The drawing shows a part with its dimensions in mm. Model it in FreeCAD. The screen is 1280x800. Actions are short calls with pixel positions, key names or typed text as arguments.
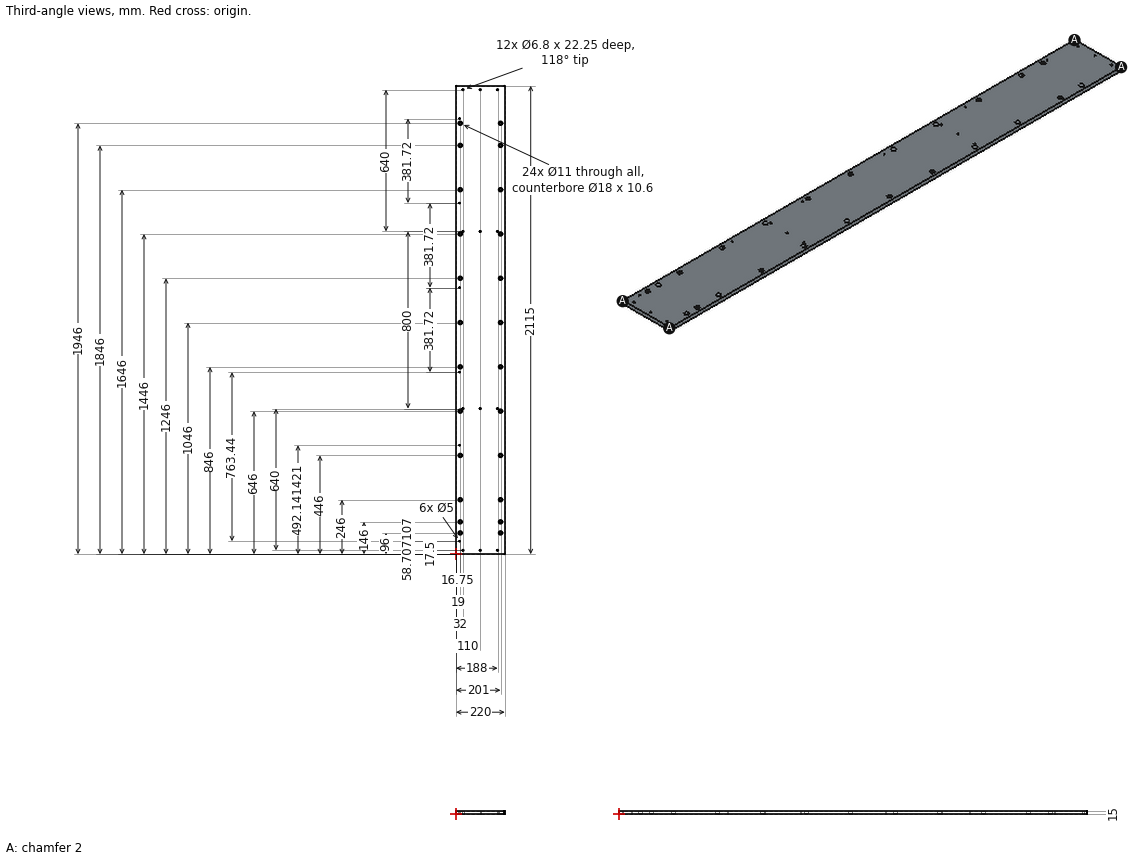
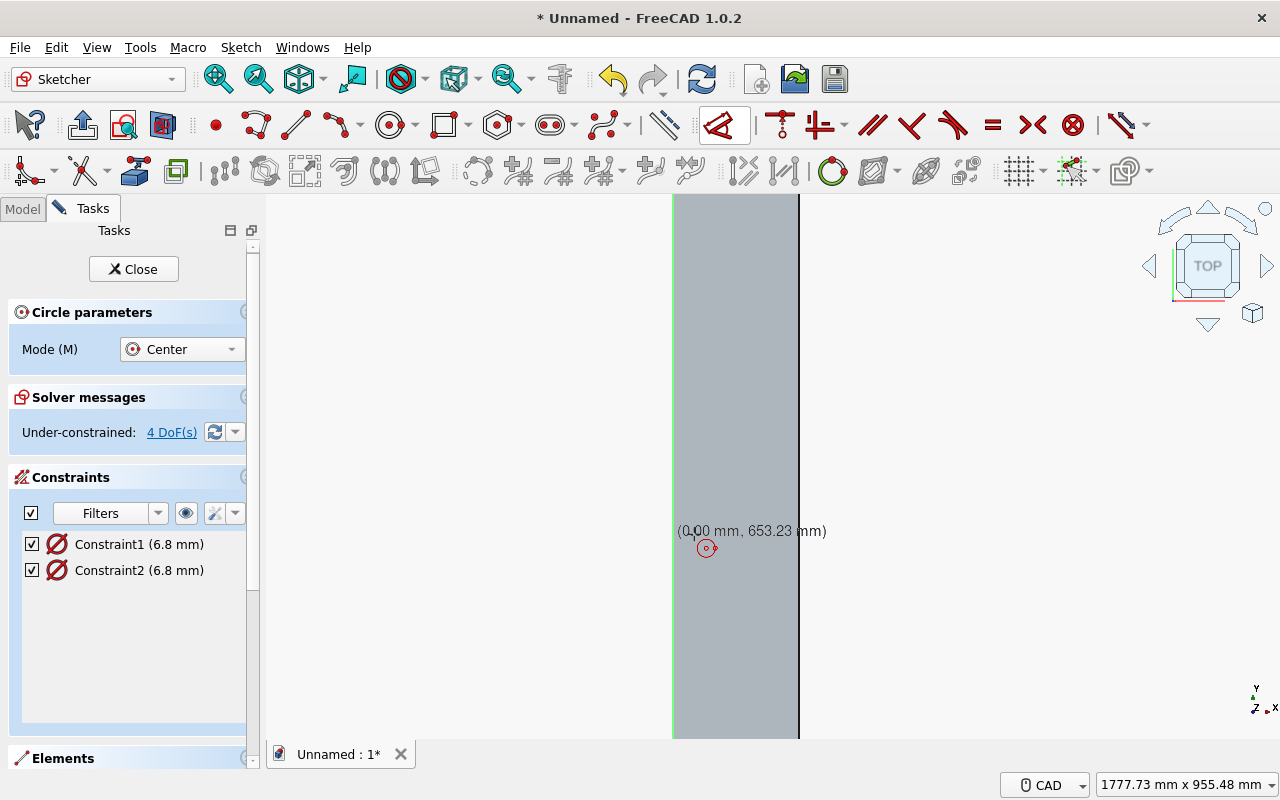
click(692, 533)
move(693, 532)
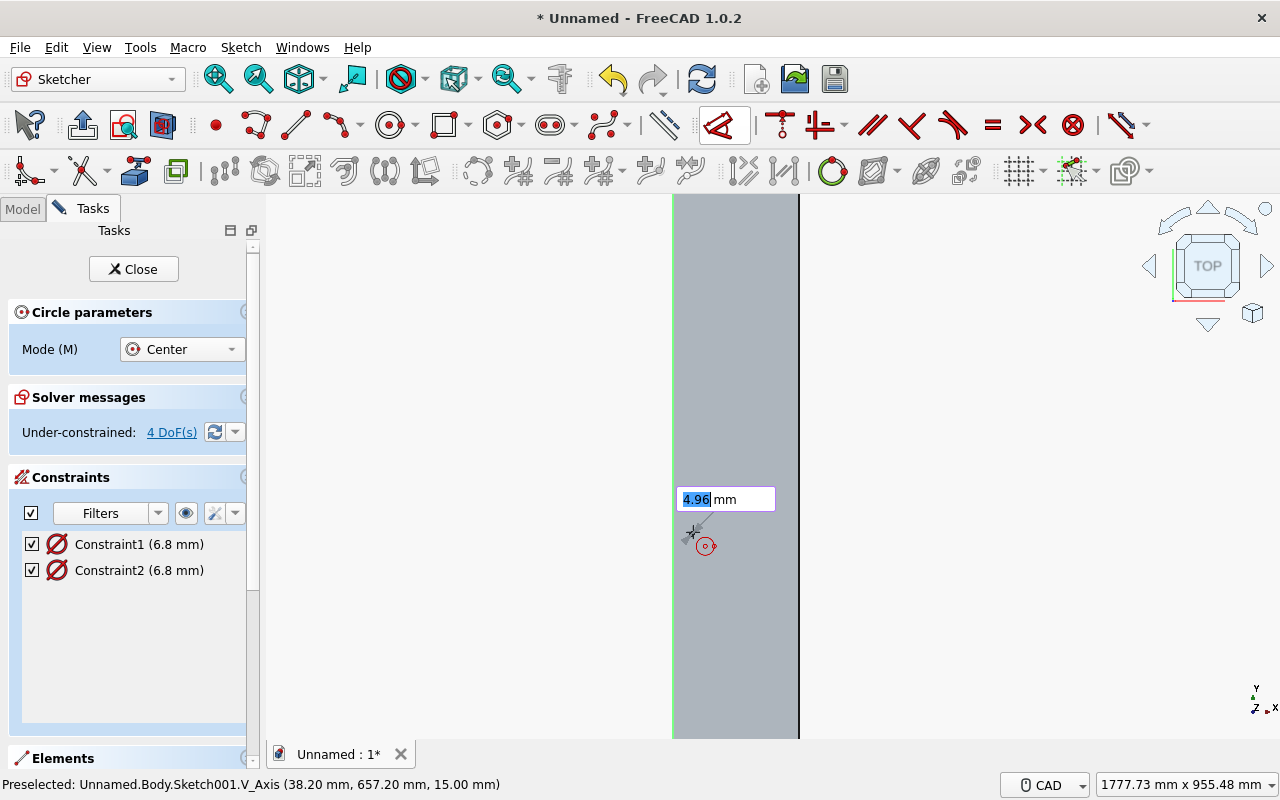
text(6.8)
key(Return)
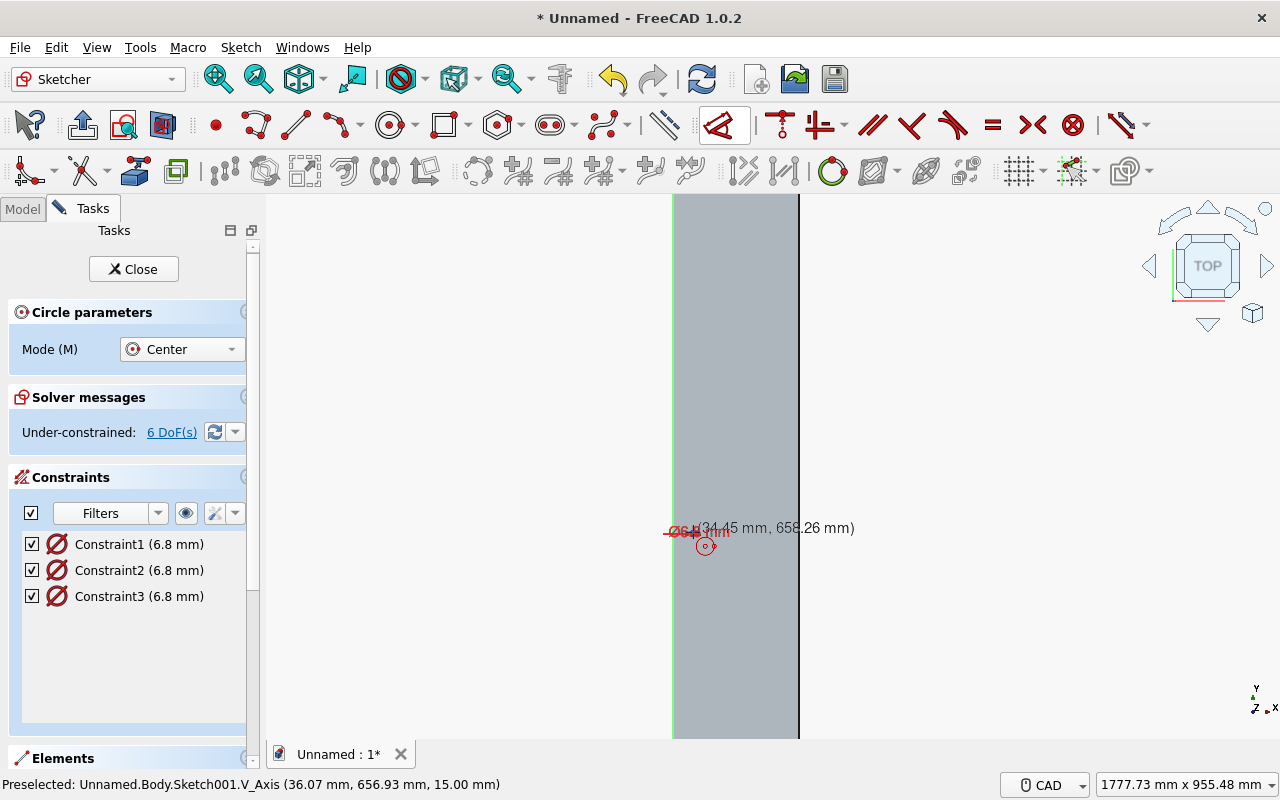
scroll(694, 534, down, 6)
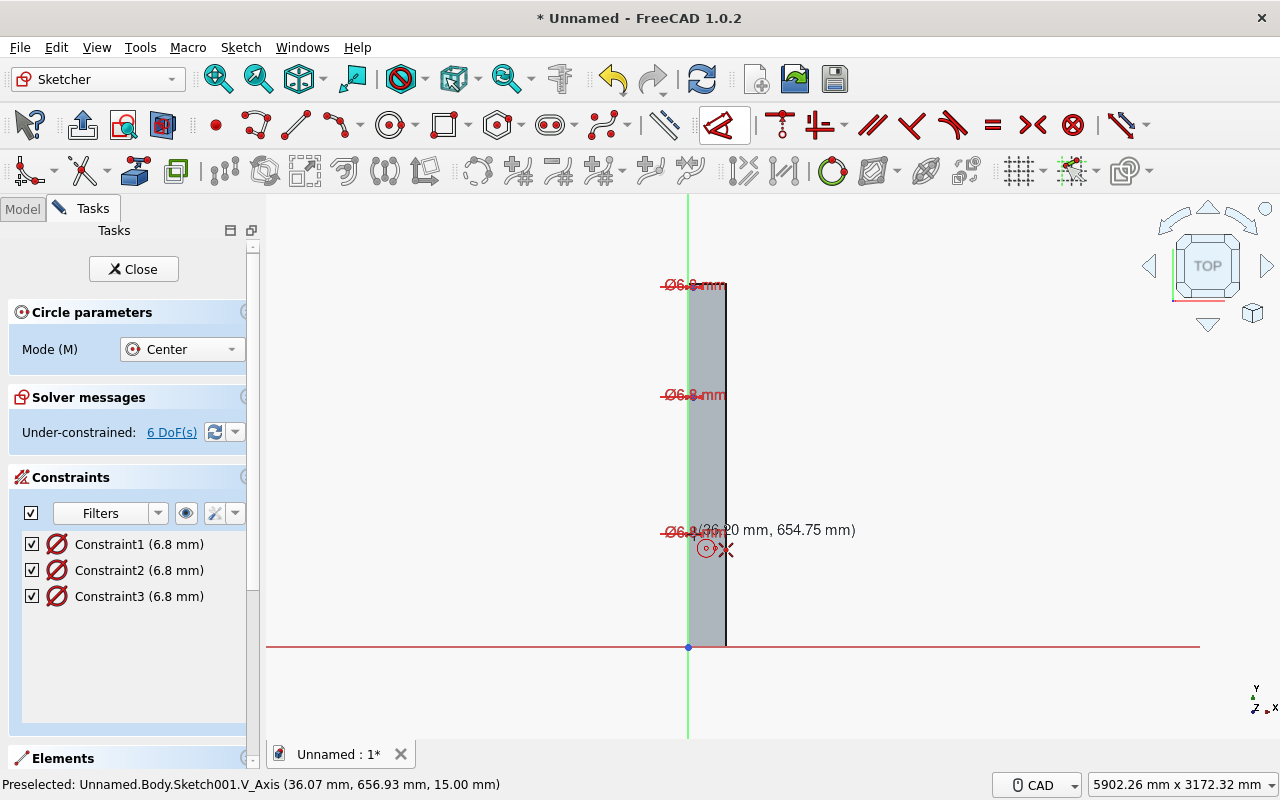
scroll(694, 644, up, 19)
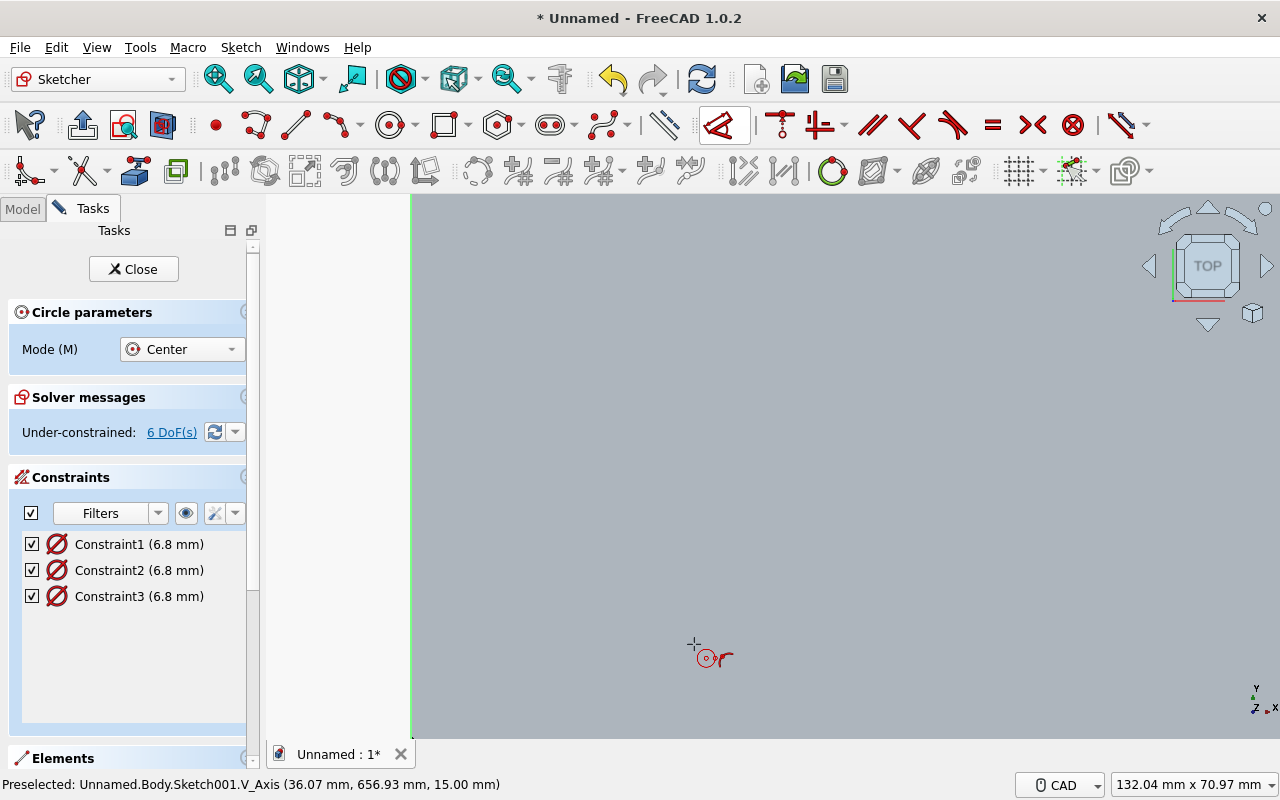
scroll(704, 466, down, 15)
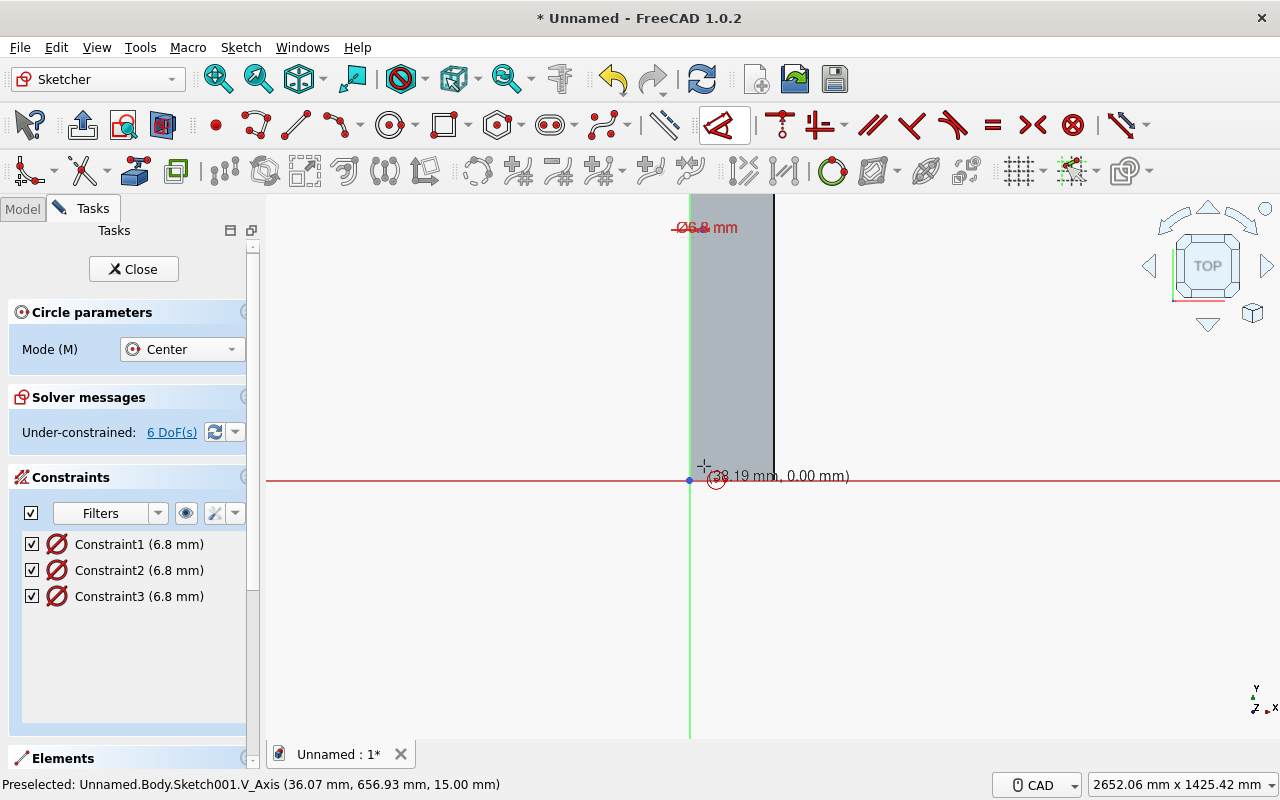
scroll(692, 692, down, 5)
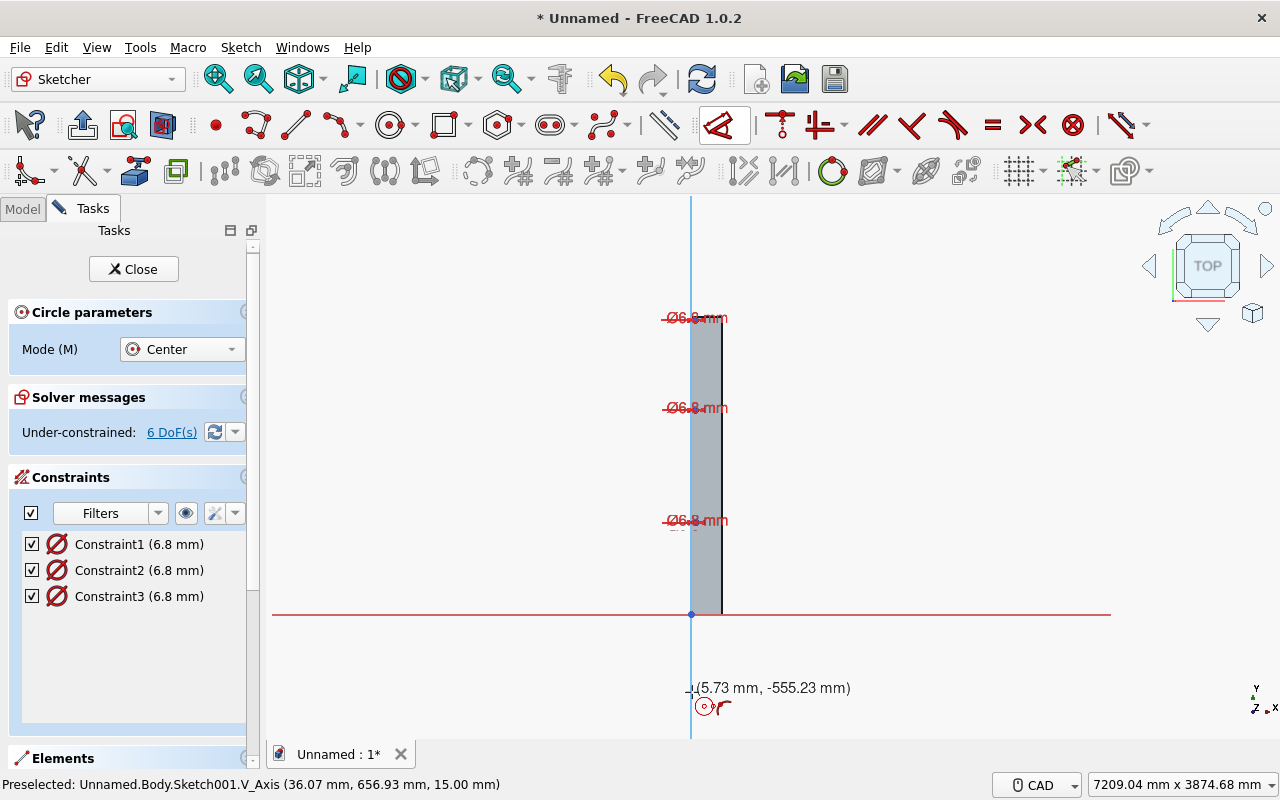
scroll(696, 612, up, 10)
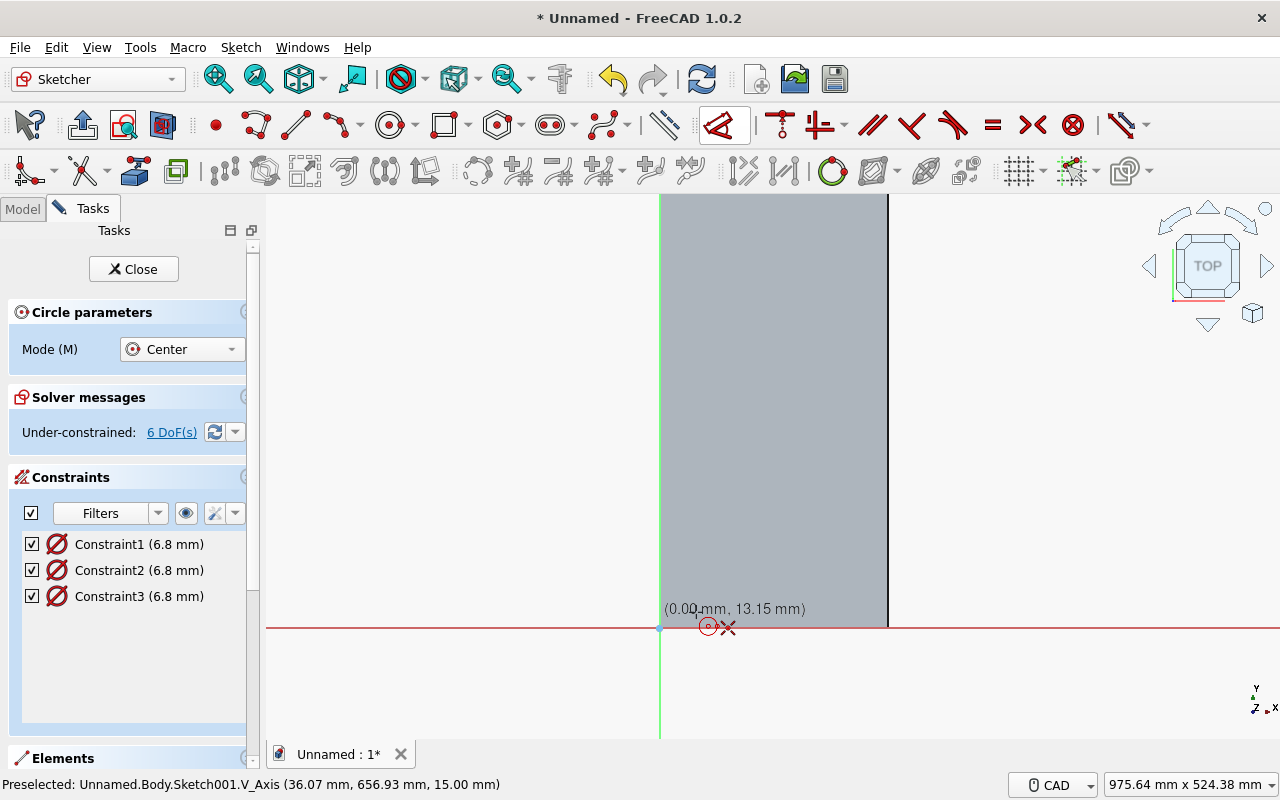
click(693, 610)
move(695, 607)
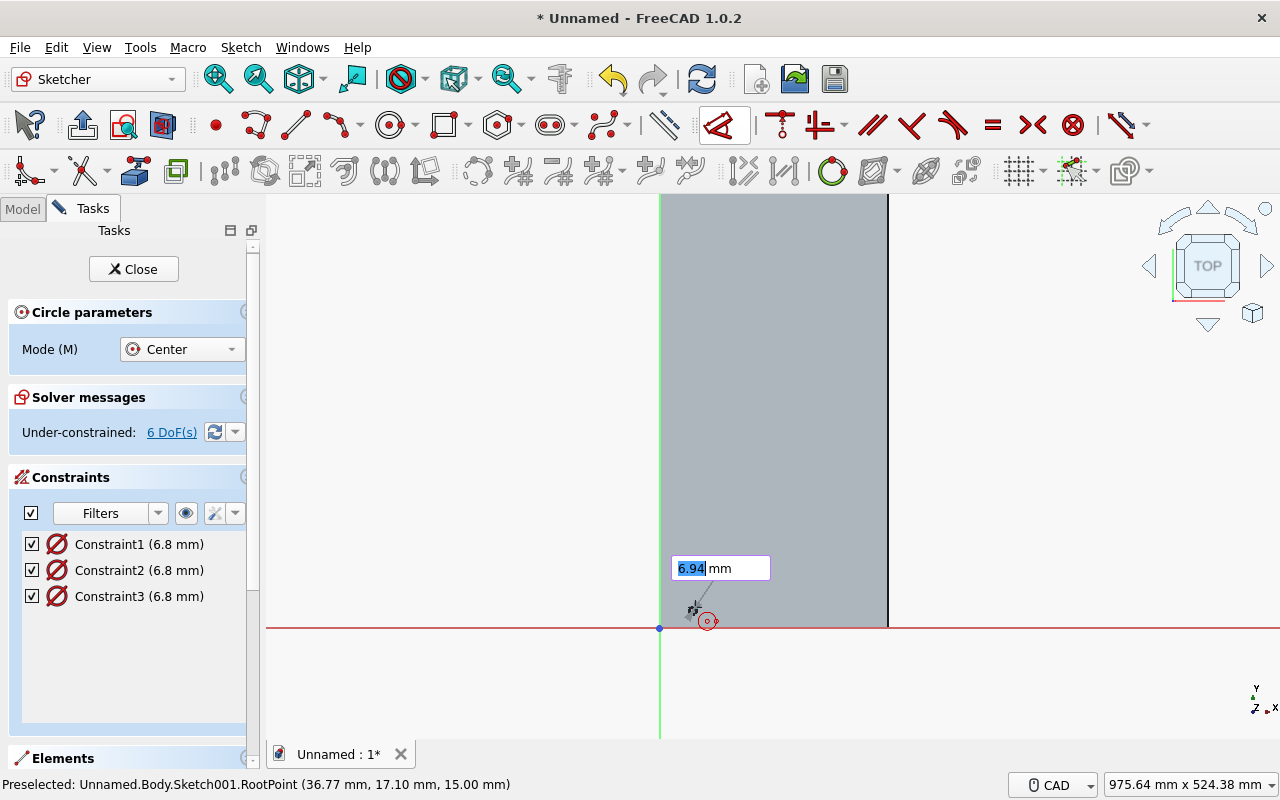
text(6.8)
key(Return)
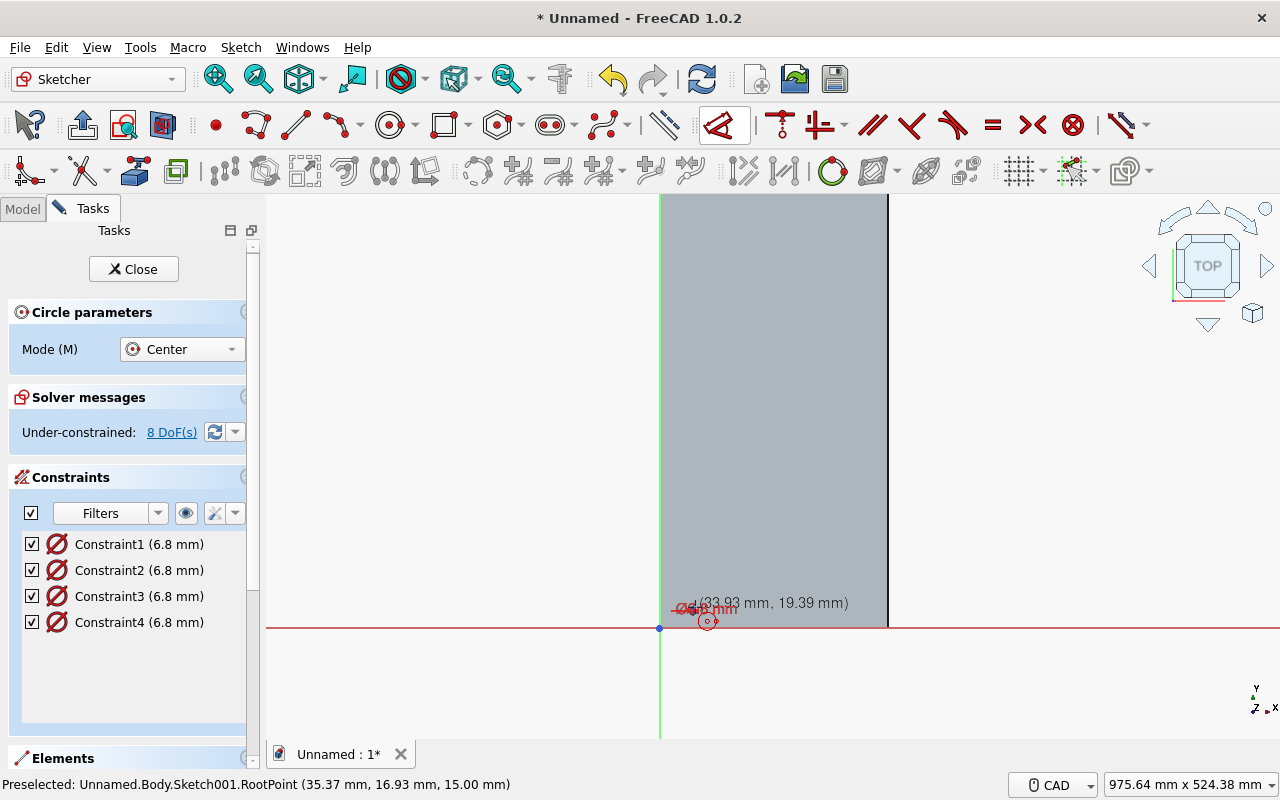
scroll(694, 651, down, 9)